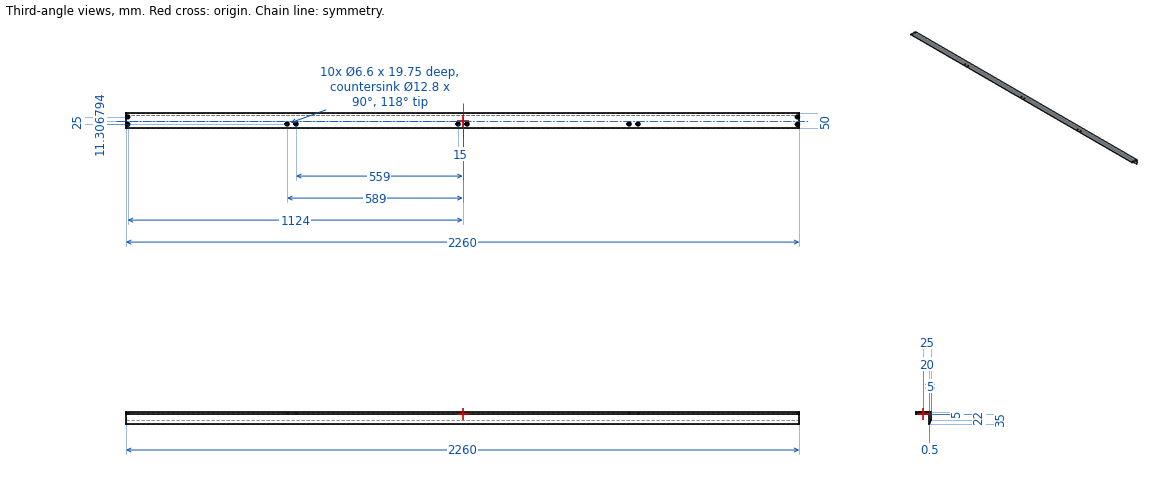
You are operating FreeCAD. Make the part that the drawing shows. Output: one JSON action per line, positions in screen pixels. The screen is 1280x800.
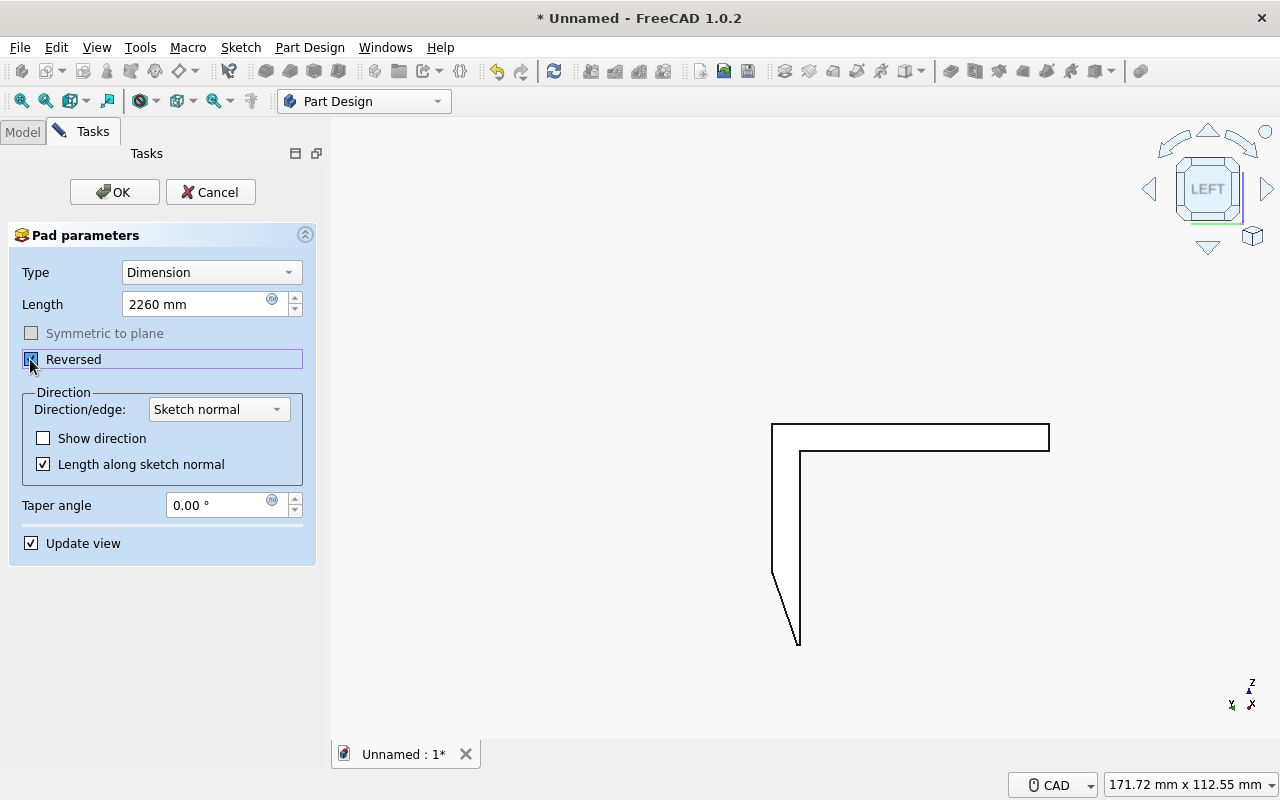
{"action": "left_click", "coordinate": [115, 192]}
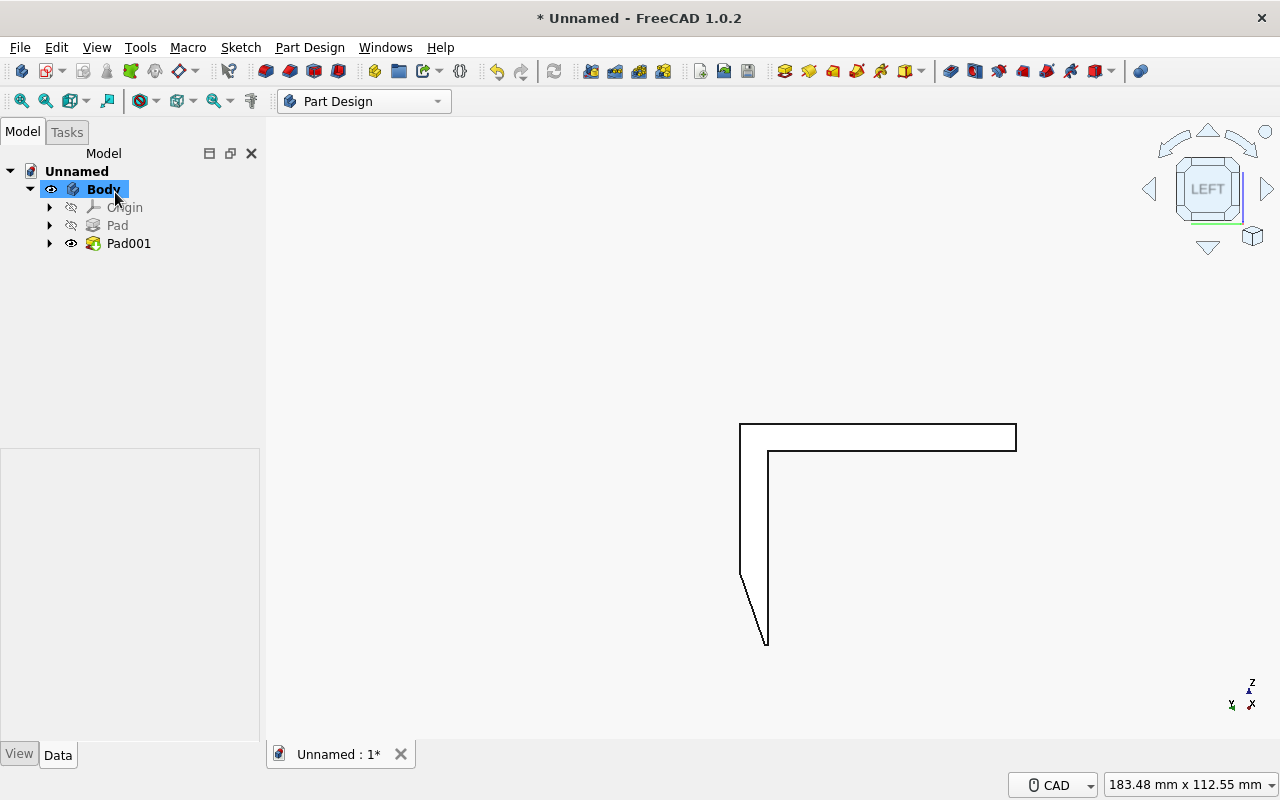
{"action": "left_click", "coordinate": [22, 102]}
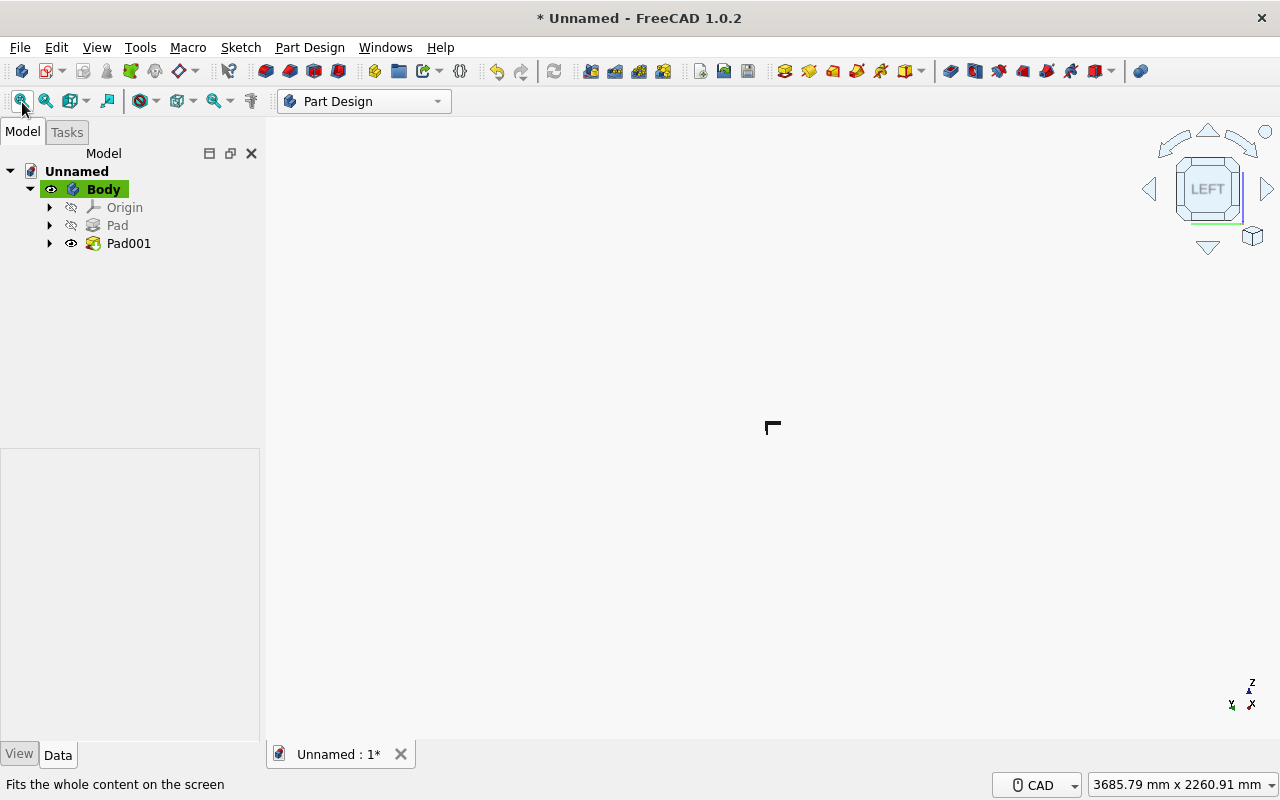
{"action": "key", "text": "0"}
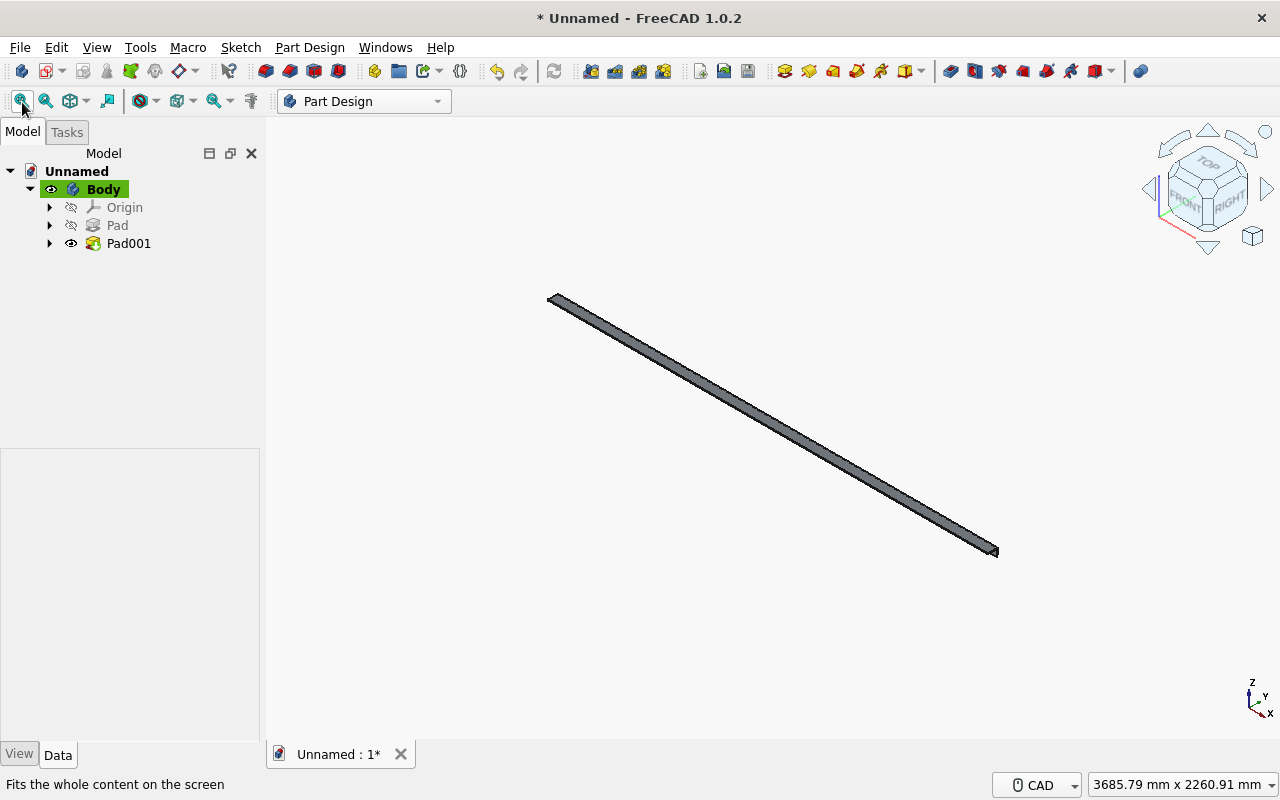
{"action": "left_click", "coordinate": [22, 102]}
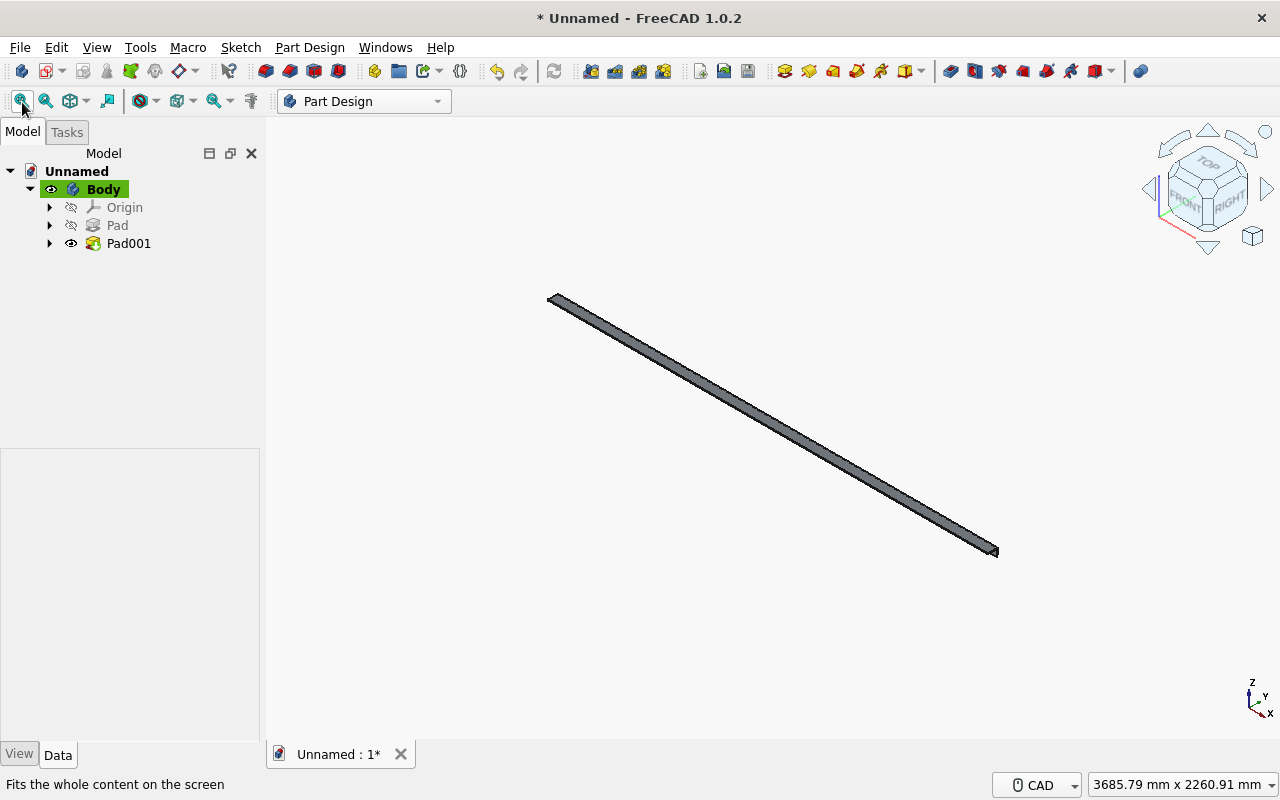
{"action": "scroll", "coordinate": [961, 531], "scroll_direction": "up", "scroll_amount": 3}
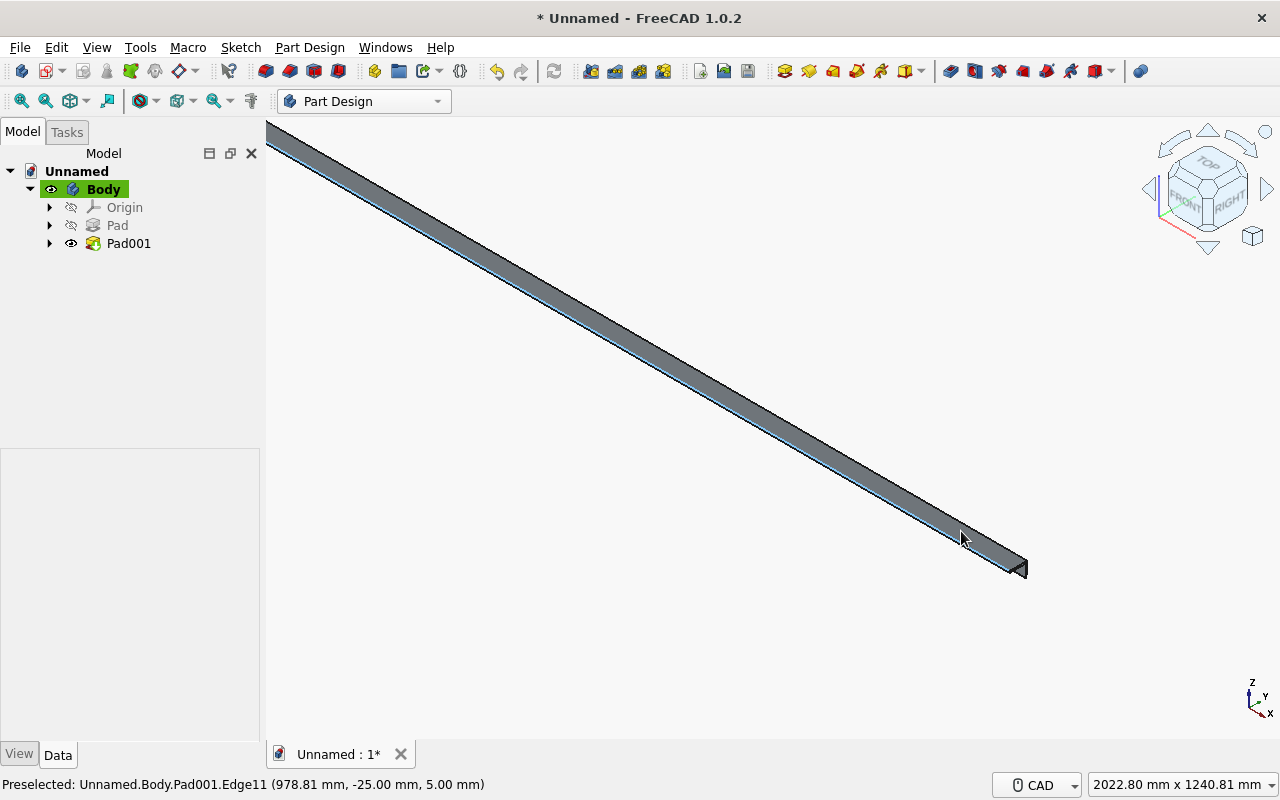
{"action": "left_click", "coordinate": [389, 201]}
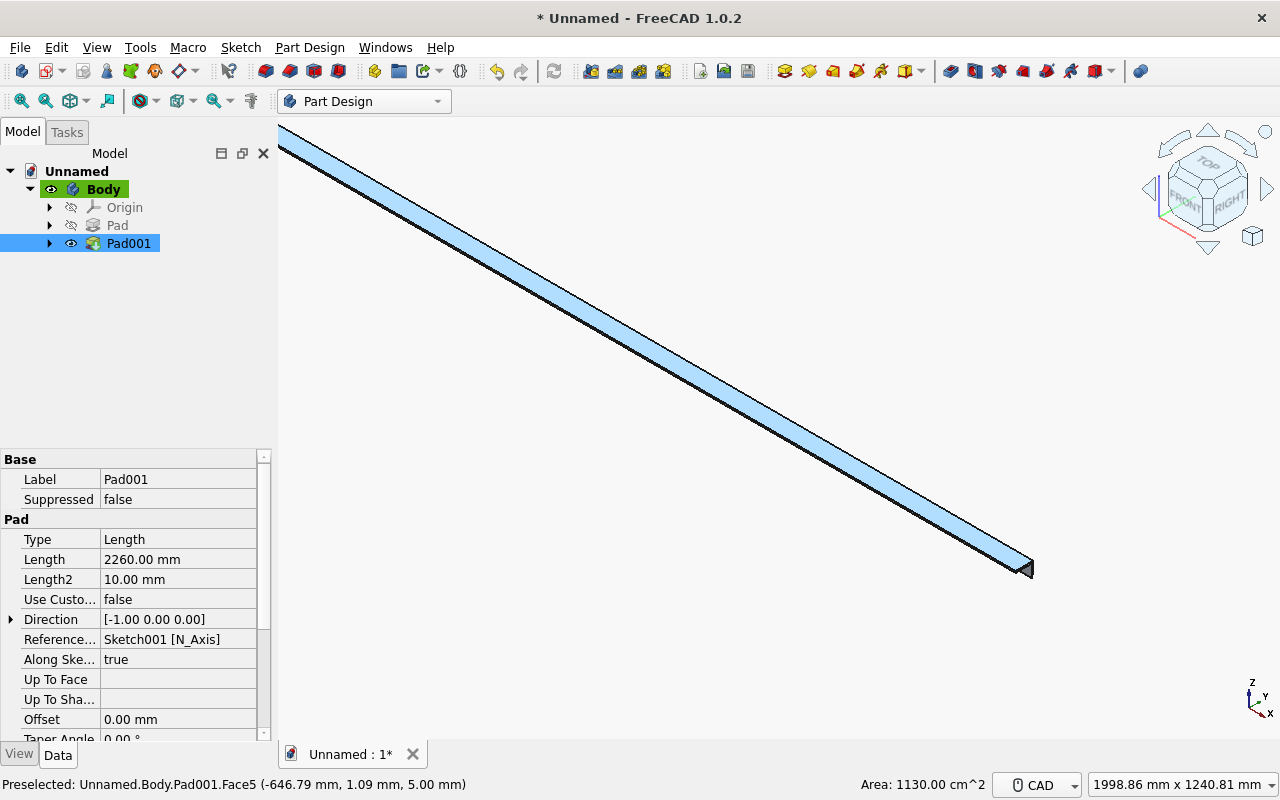
{"action": "left_click", "coordinate": [46, 72]}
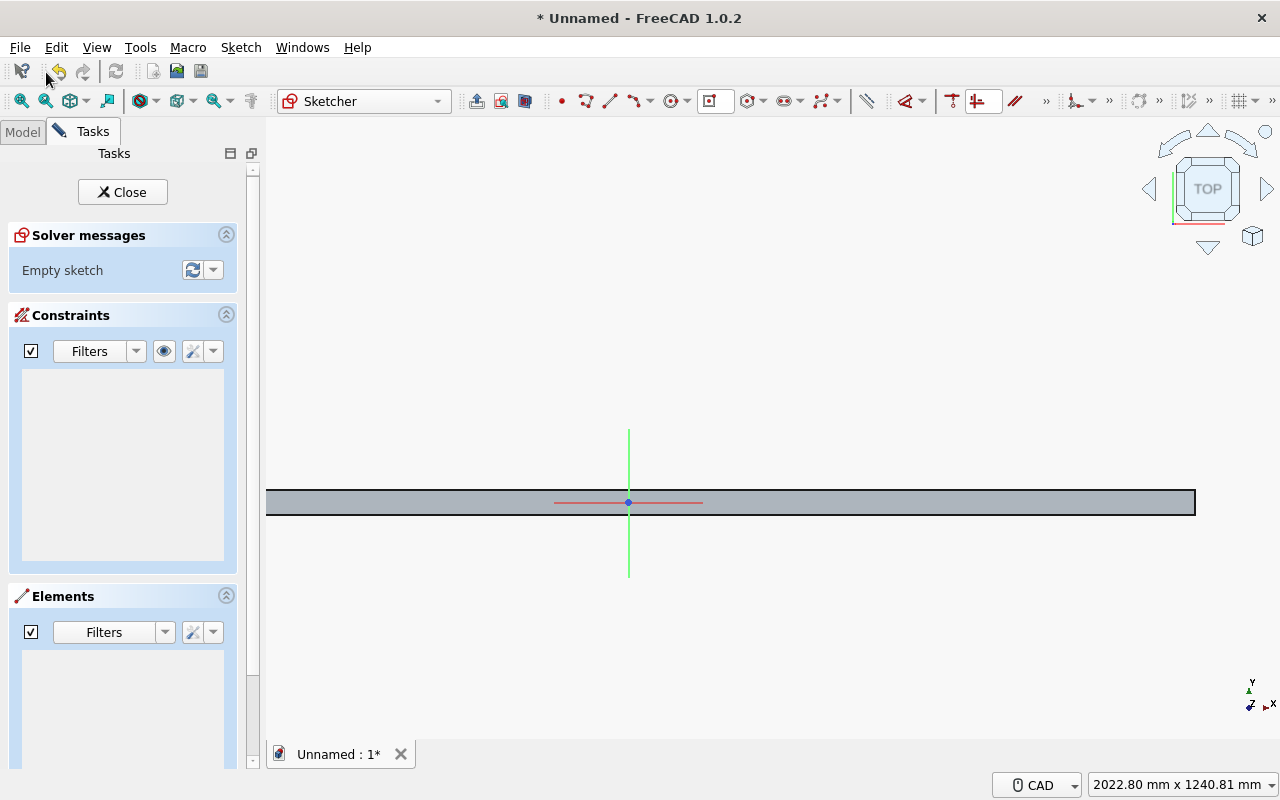
{"action": "scroll", "coordinate": [797, 337], "scroll_direction": "down", "scroll_amount": 3}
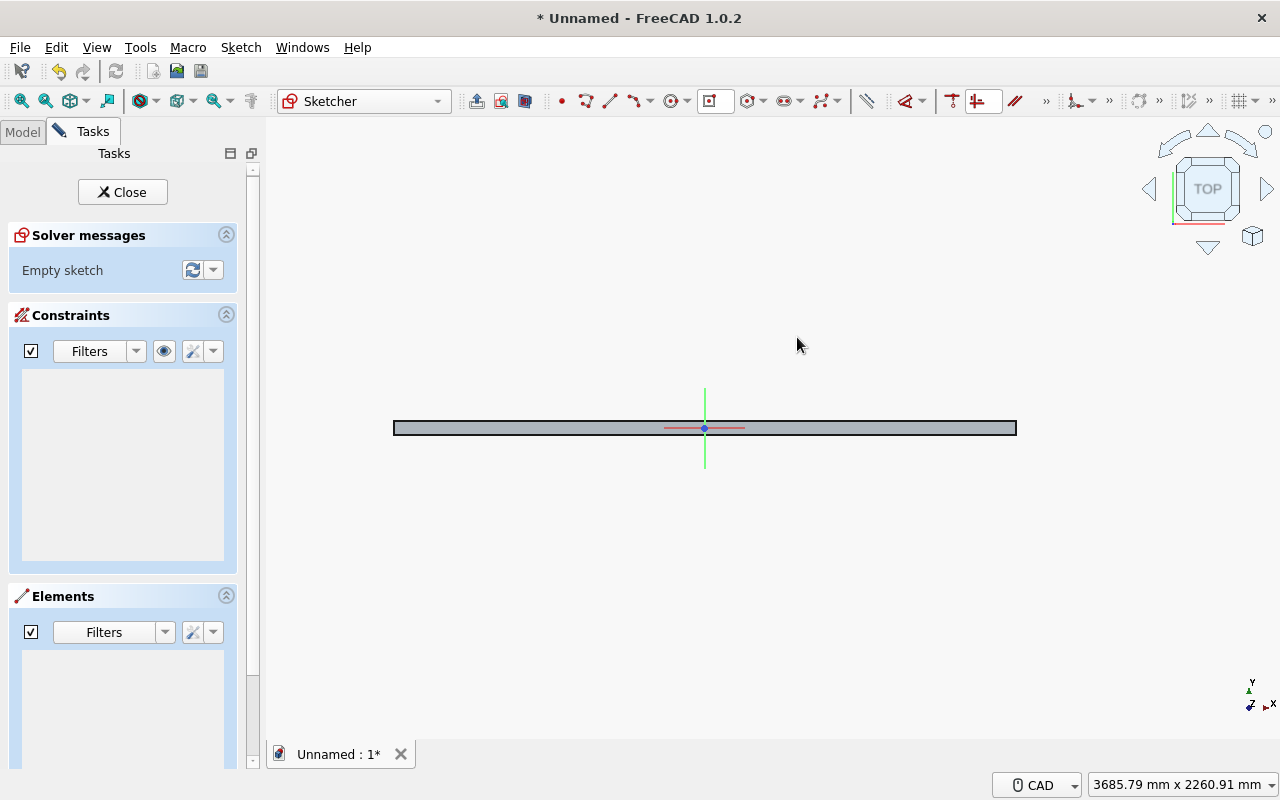
{"action": "left_click", "coordinate": [672, 102]}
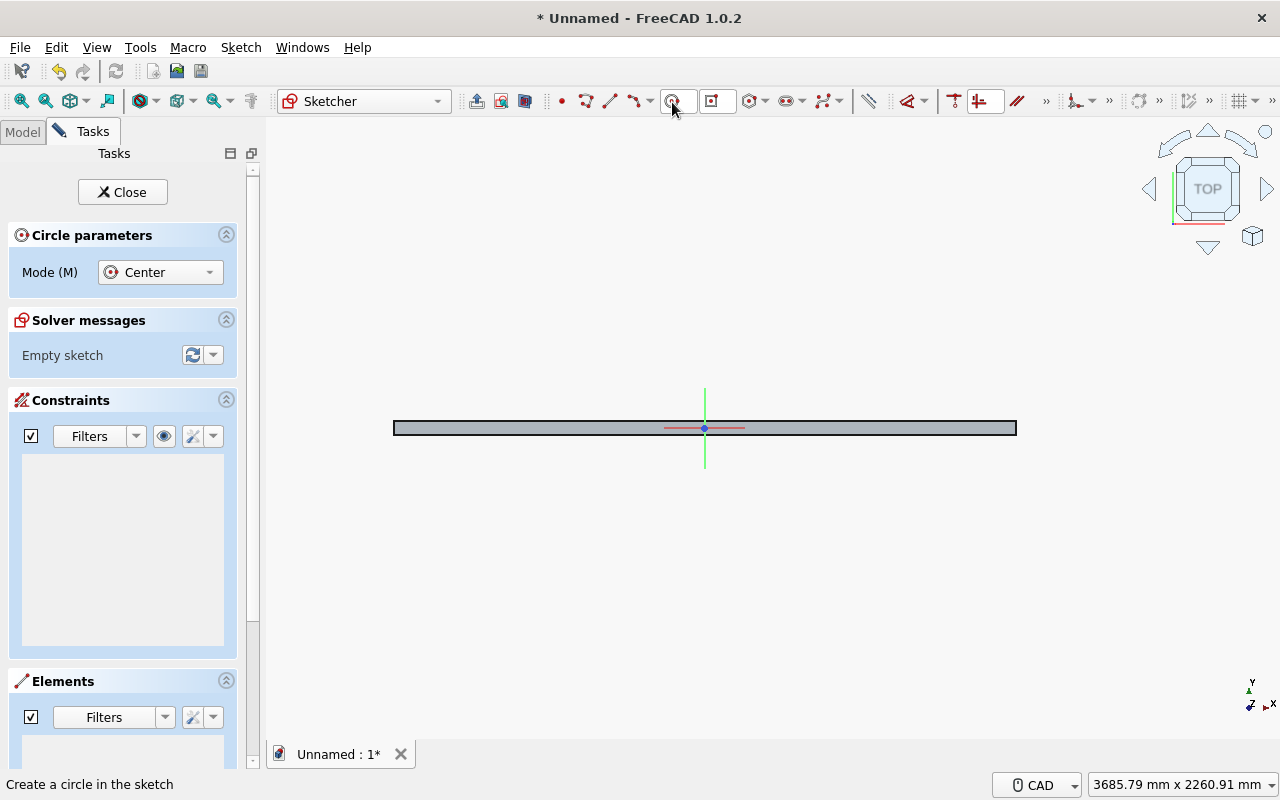
{"action": "scroll", "coordinate": [543, 431], "scroll_direction": "up", "scroll_amount": 17}